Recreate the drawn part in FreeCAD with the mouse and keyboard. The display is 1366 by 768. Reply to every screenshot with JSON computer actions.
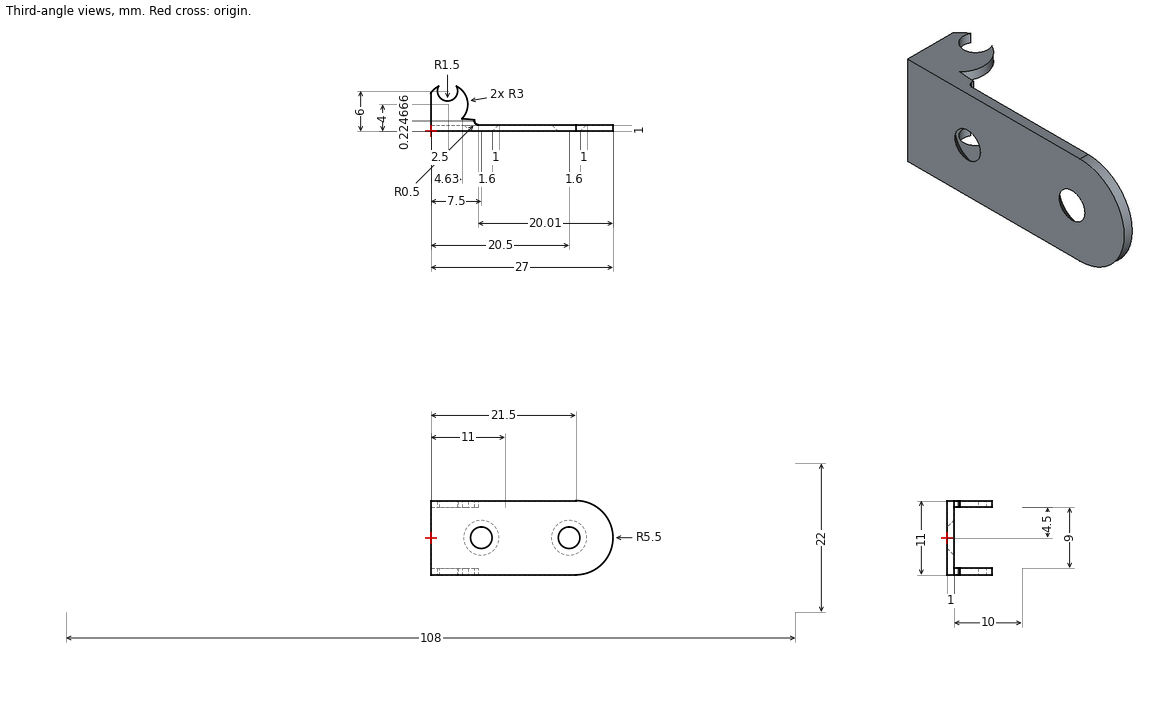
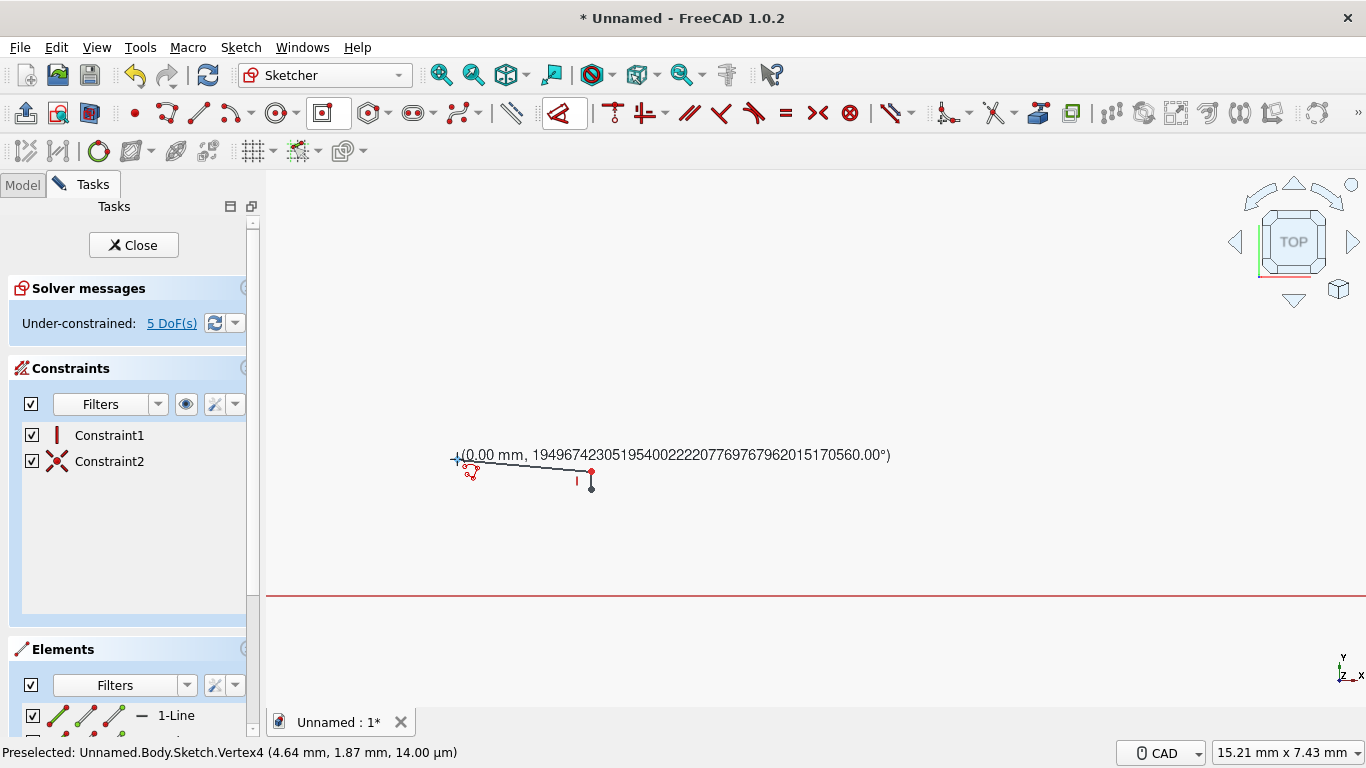
{"action": "scroll", "coordinate": [597, 475], "scroll_direction": "down", "scroll_amount": 6}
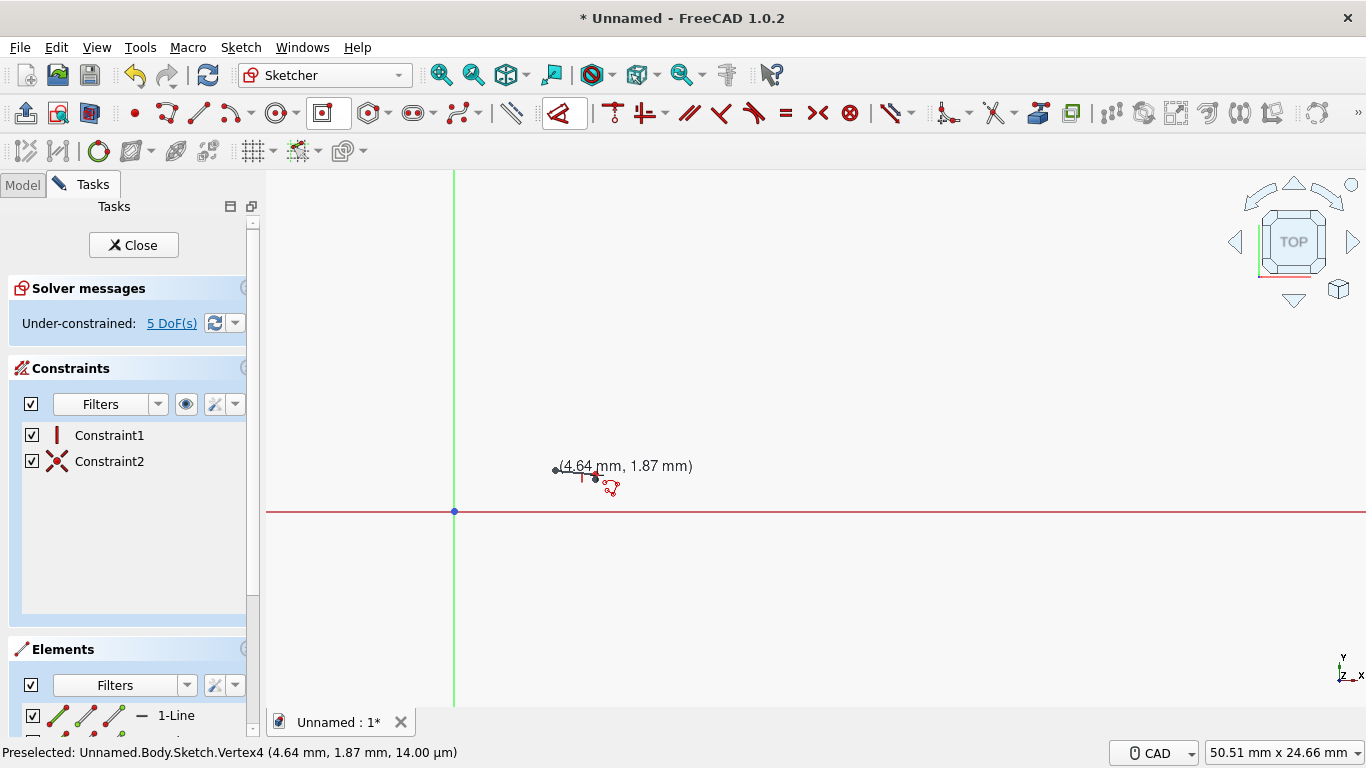
{"action": "left_click", "coordinate": [454, 388]}
{"action": "left_click", "coordinate": [454, 512]}
{"action": "left_click", "coordinate": [1042, 503]}
{"action": "left_click", "coordinate": [1042, 490]}
{"action": "left_click", "coordinate": [606, 490]}
{"action": "right_click", "coordinate": [606, 490]}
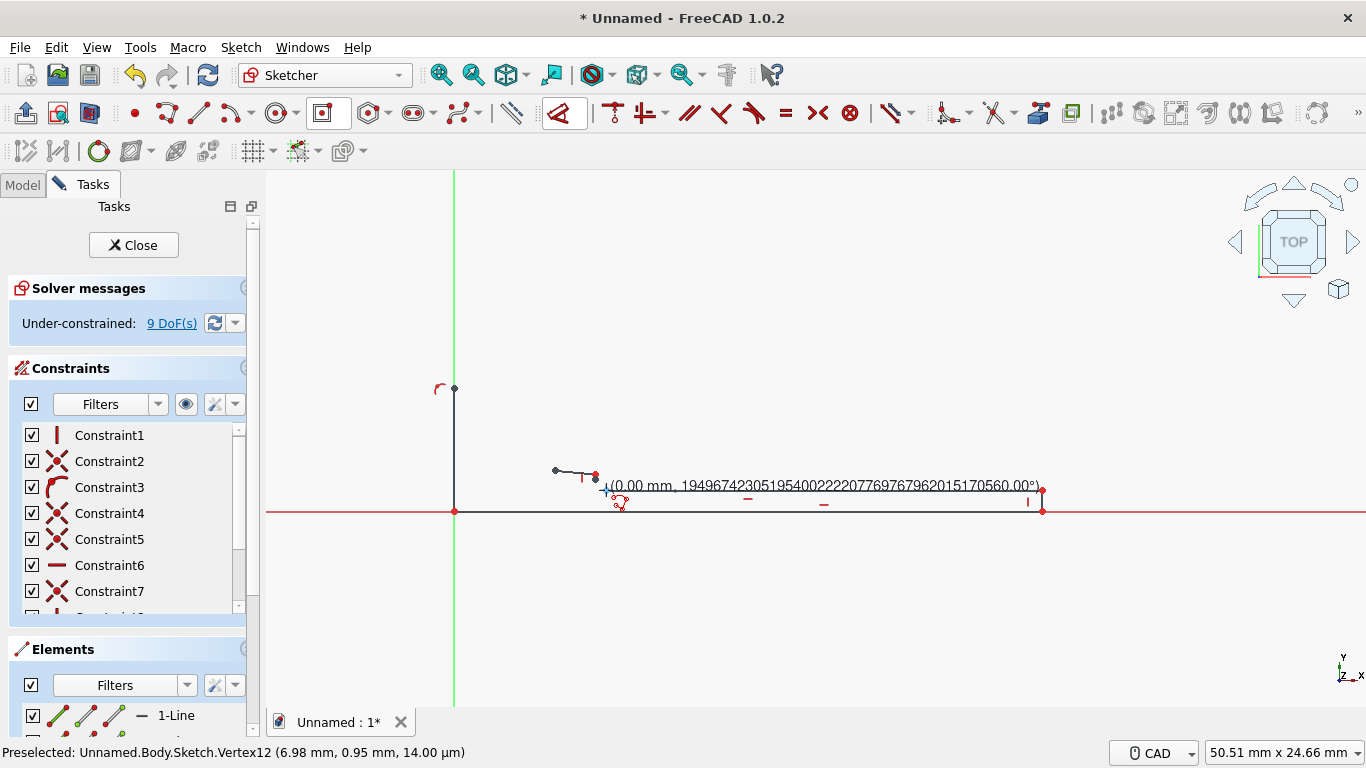
{"action": "key", "text": "g 3 a"}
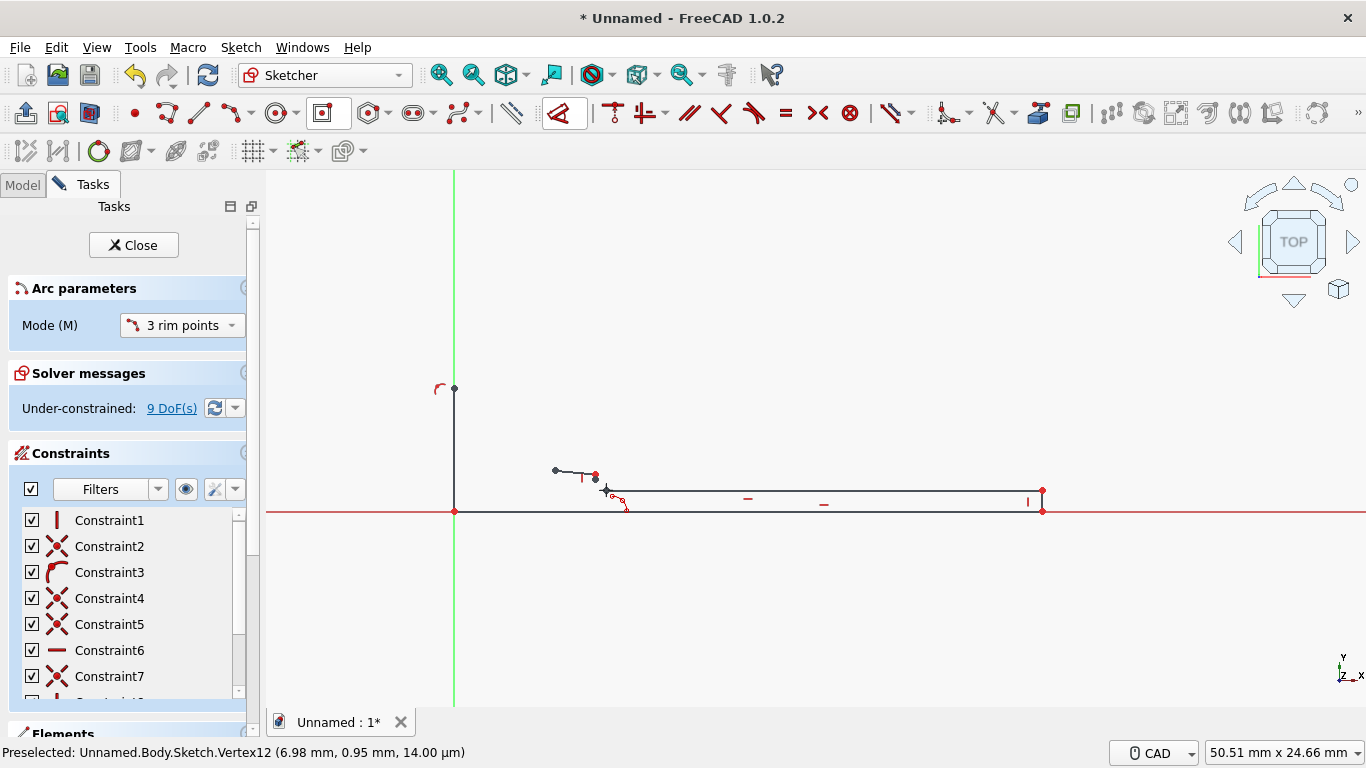
{"action": "left_click", "coordinate": [555, 471]}
{"action": "left_click", "coordinate": [538, 366]}
{"action": "left_click", "coordinate": [573, 414]}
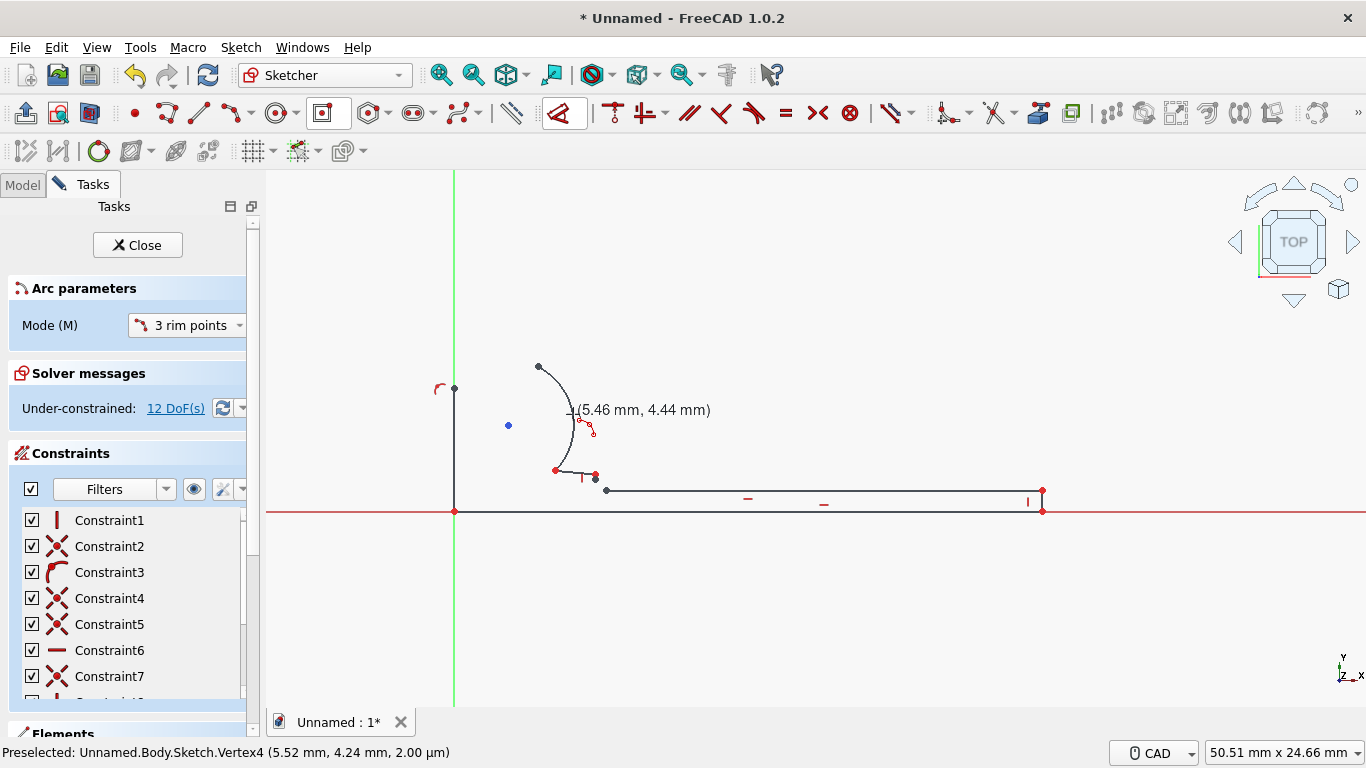
{"action": "left_click", "coordinate": [538, 367]}
{"action": "left_click", "coordinate": [479, 366]}
{"action": "left_click", "coordinate": [496, 411]}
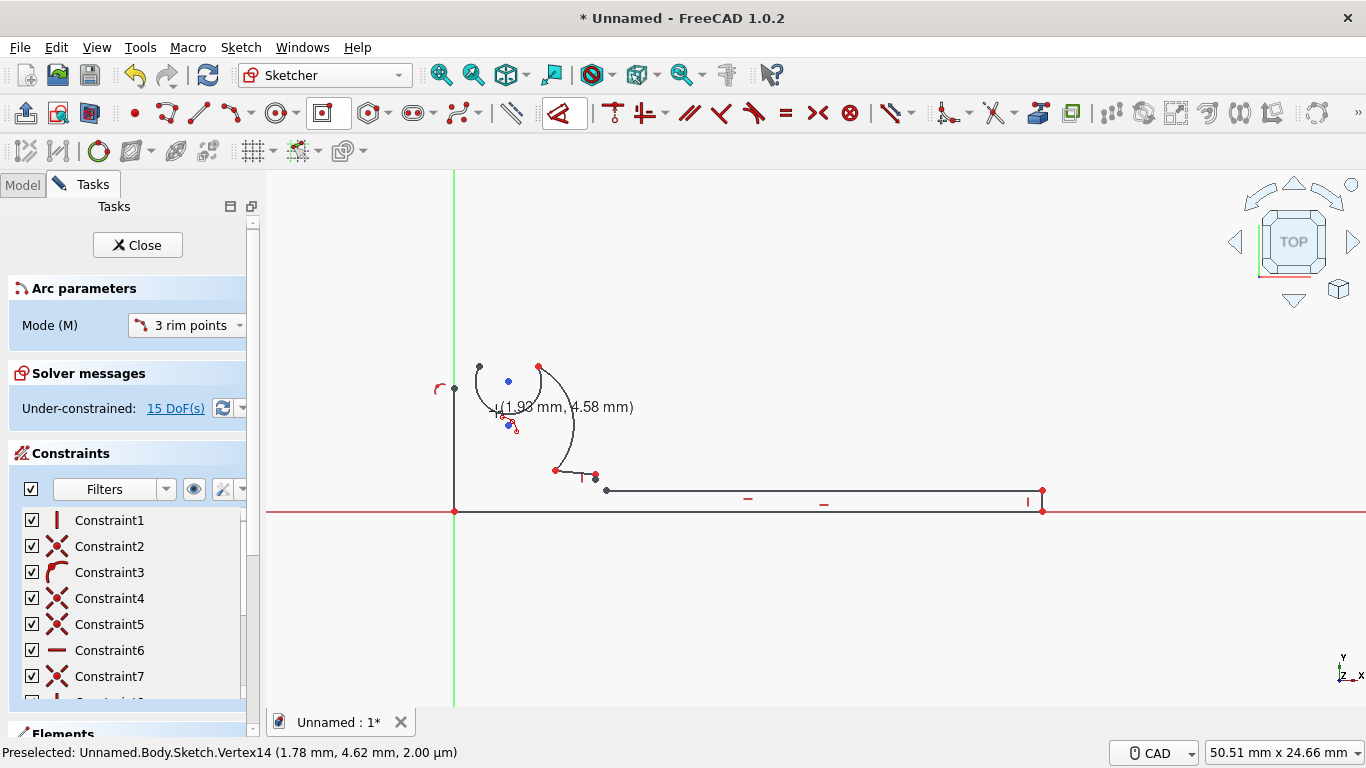
{"action": "left_click", "coordinate": [479, 367]}
{"action": "left_click", "coordinate": [454, 389]}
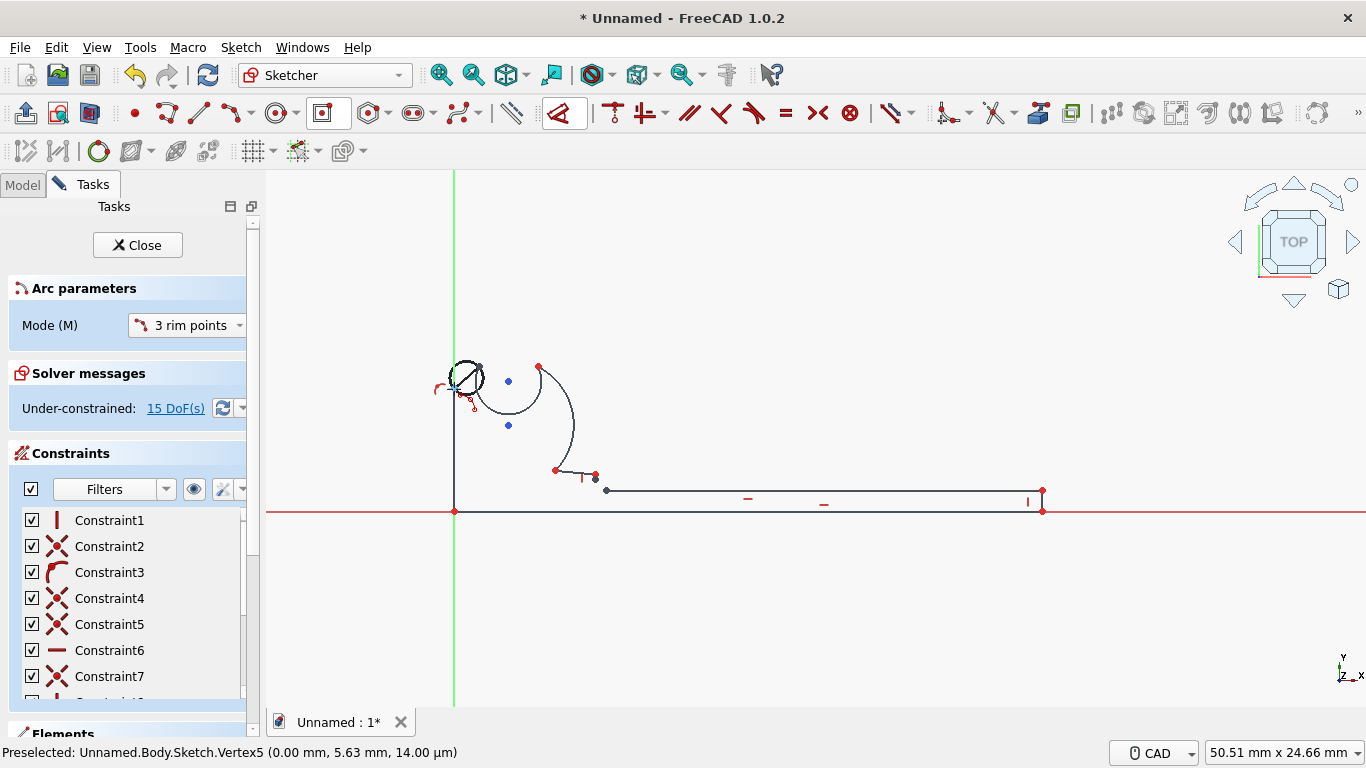
{"action": "scroll", "coordinate": [465, 376], "scroll_direction": "up", "scroll_amount": 10}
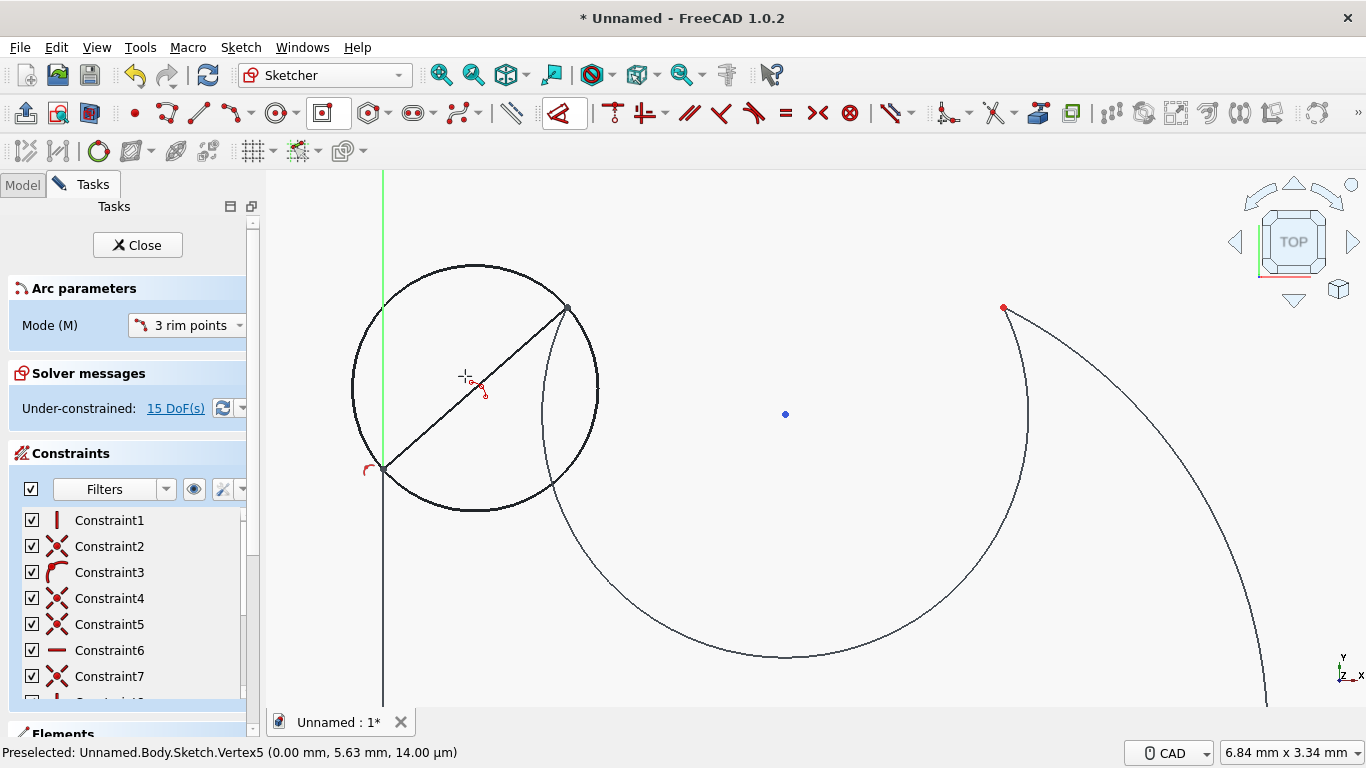
{"action": "left_click", "coordinate": [466, 371]}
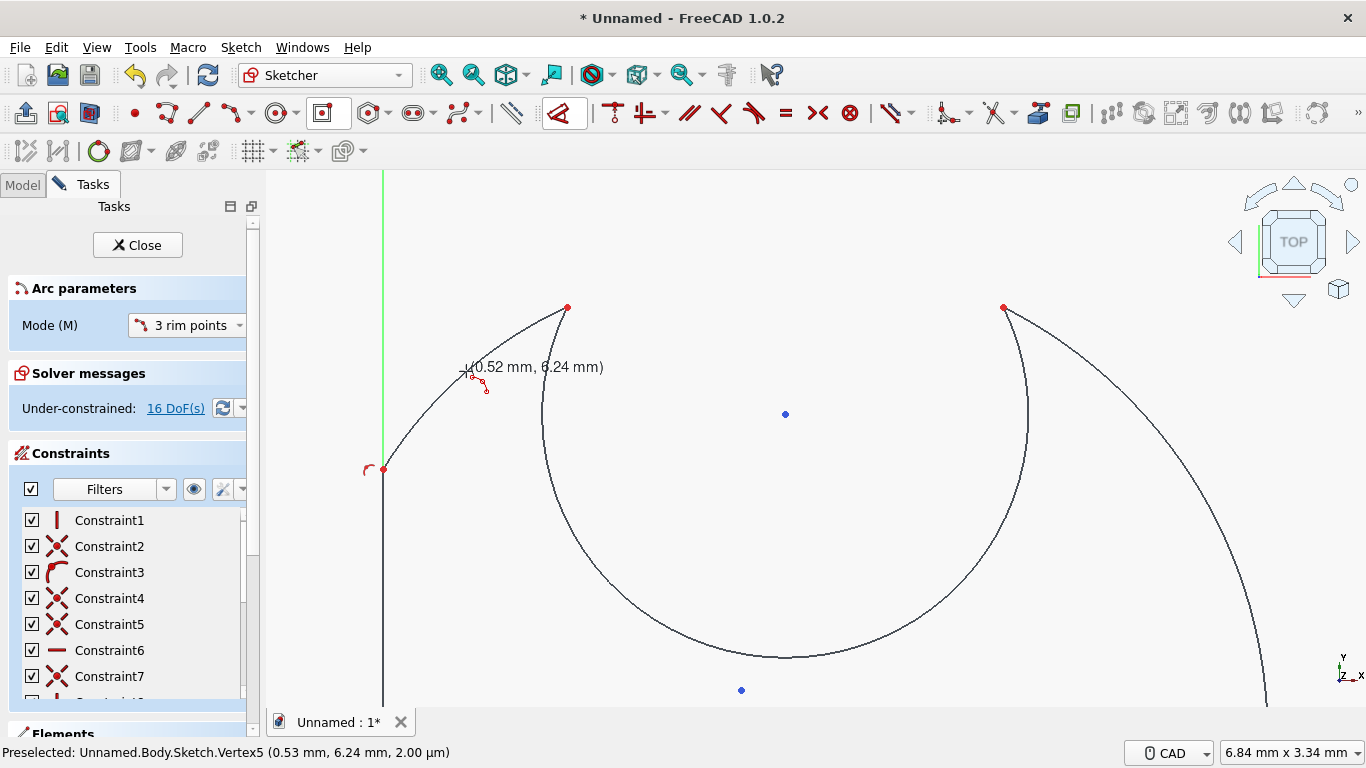
{"action": "scroll", "coordinate": [465, 376], "scroll_direction": "down", "scroll_amount": 10}